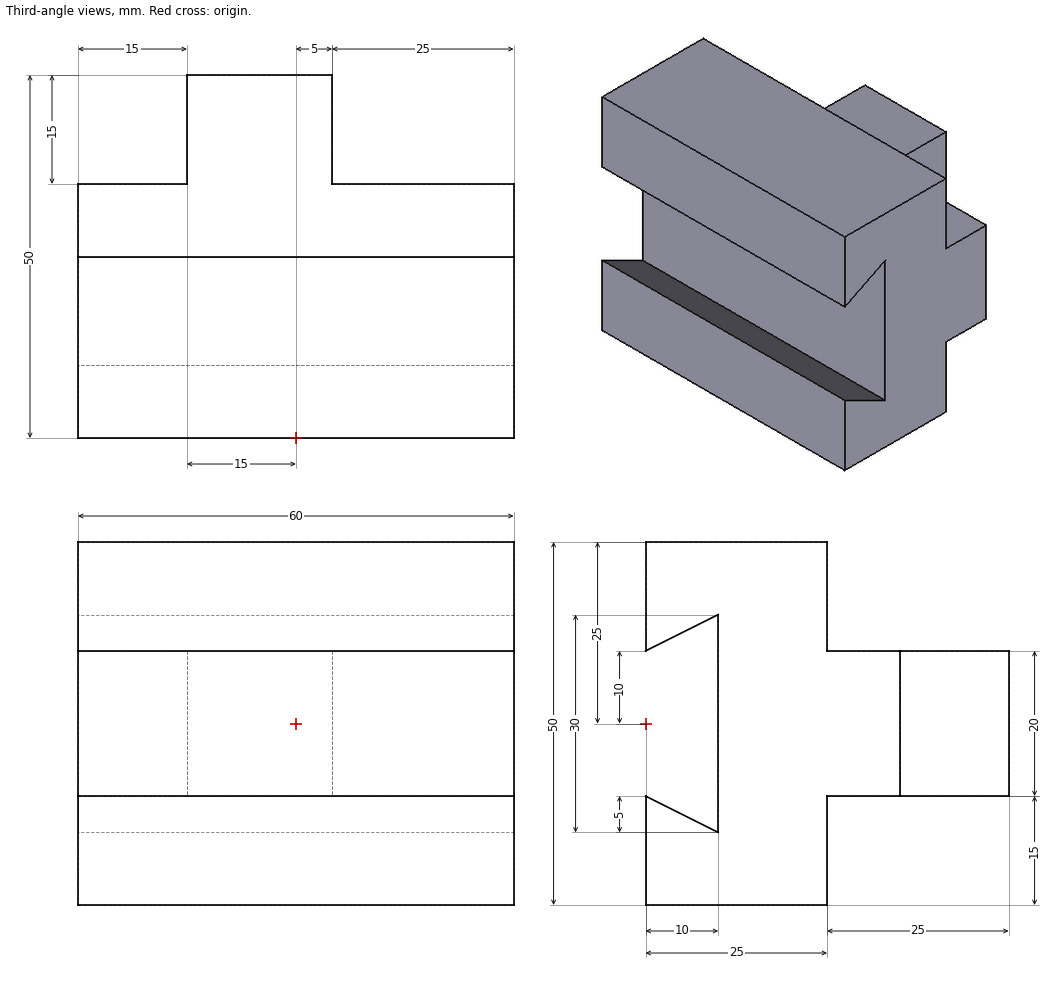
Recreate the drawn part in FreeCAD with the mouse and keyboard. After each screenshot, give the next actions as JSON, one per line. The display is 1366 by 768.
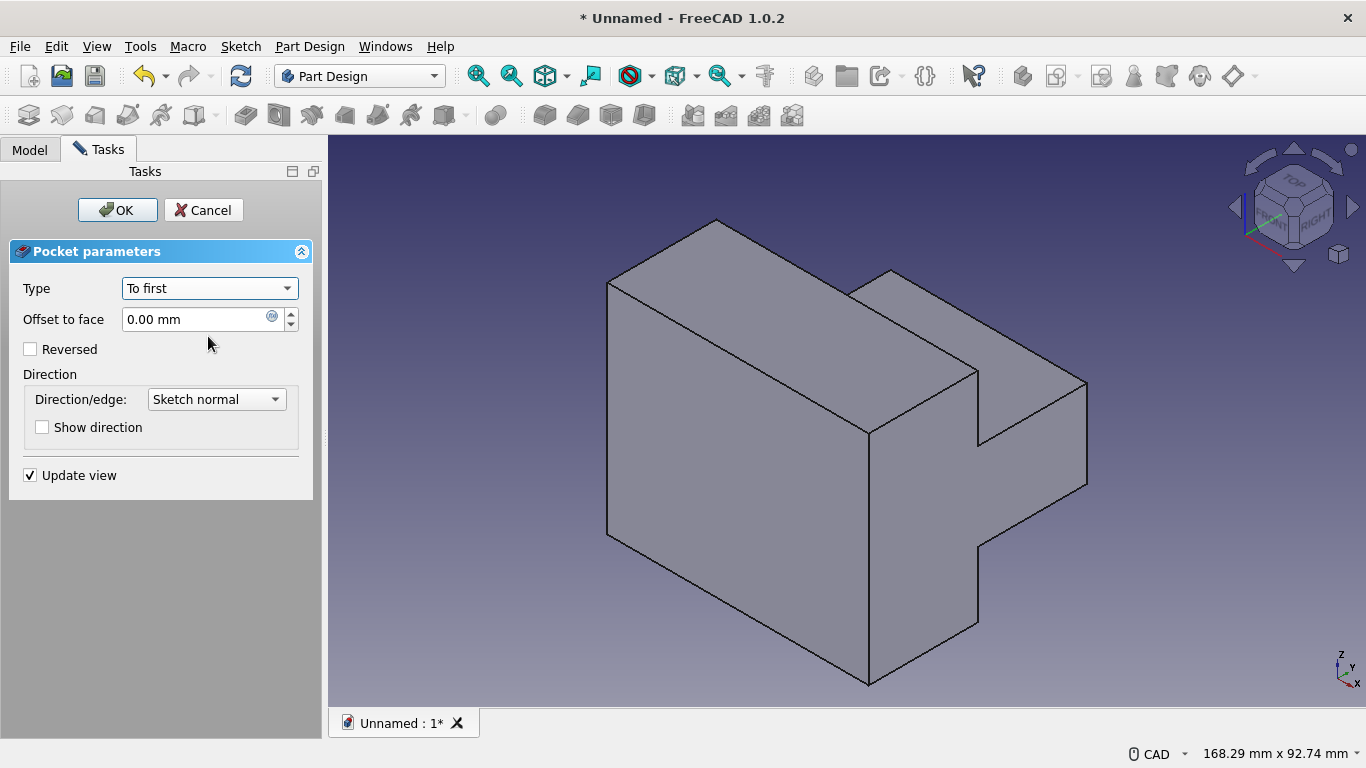
{"action": "left_click", "coordinate": [118, 210]}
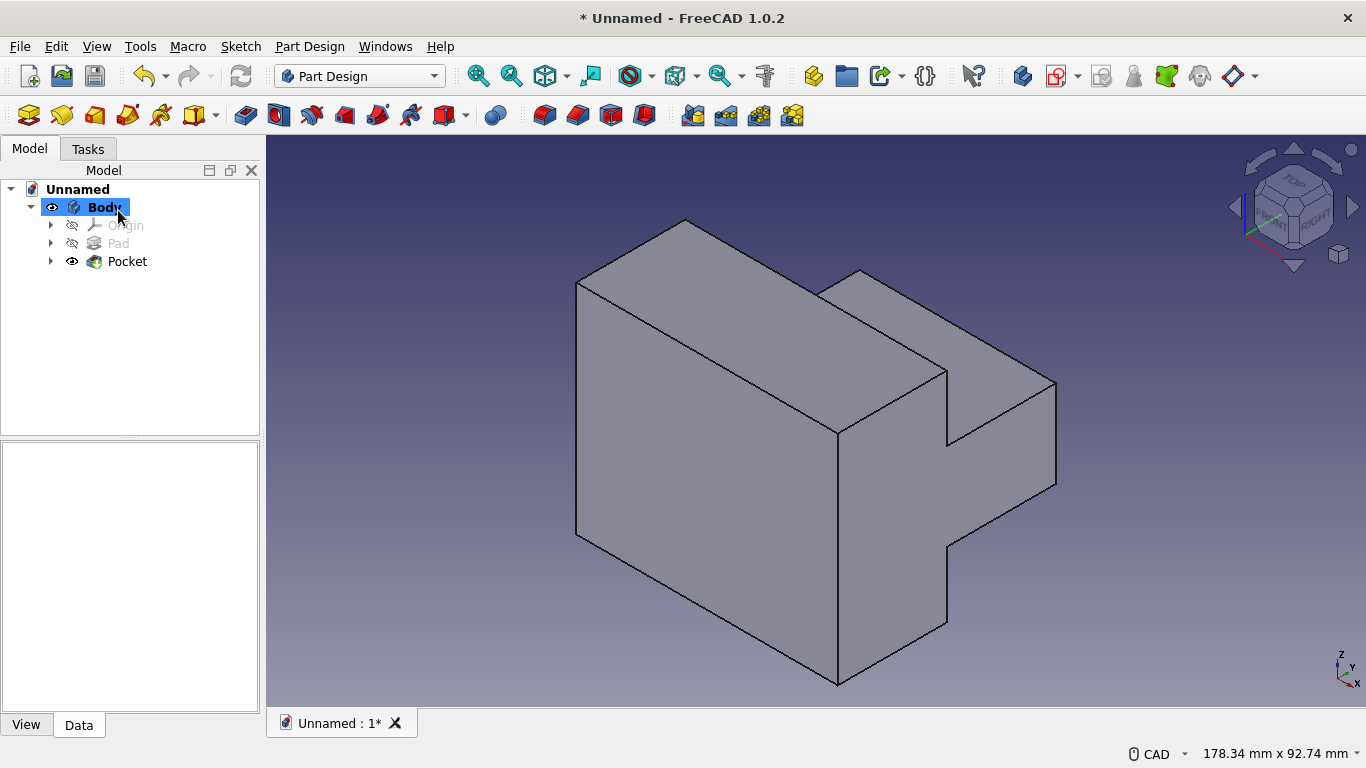
{"action": "left_click", "coordinate": [961, 372]}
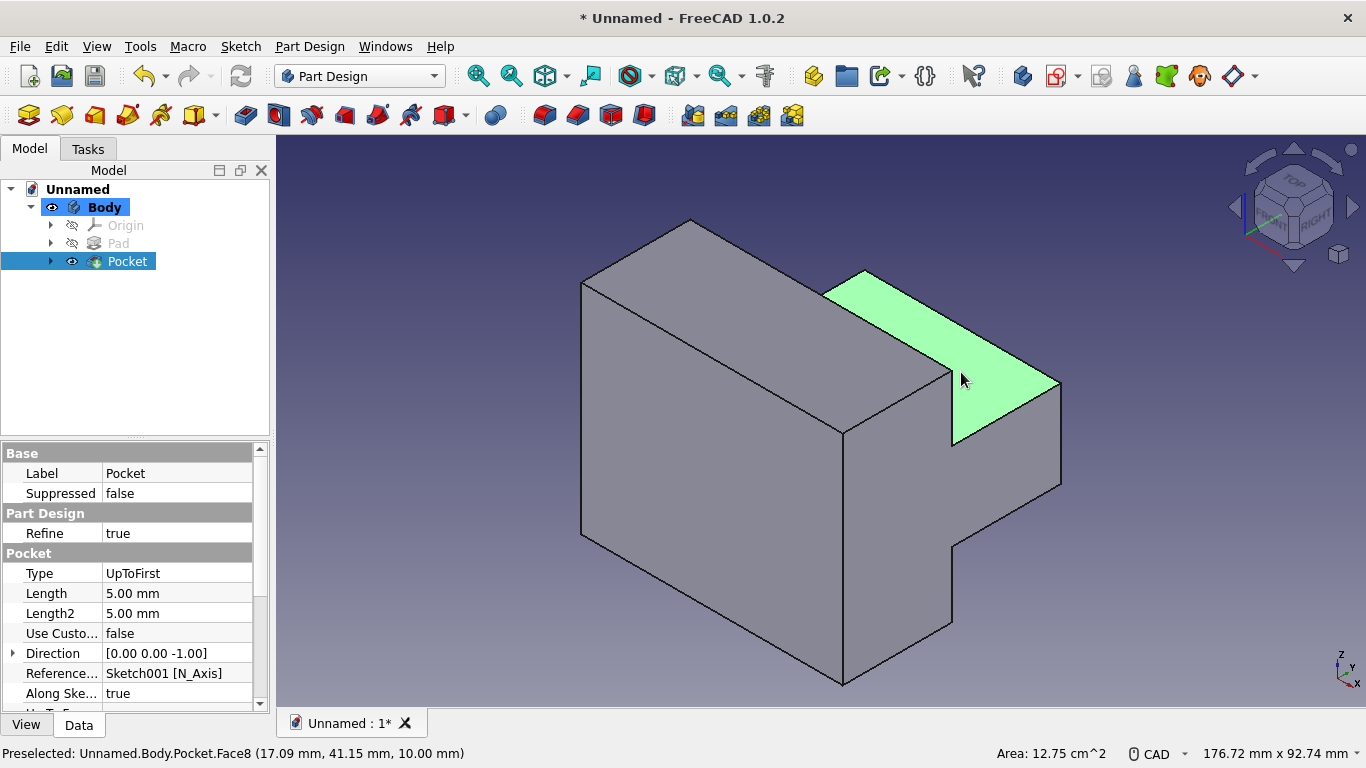
{"action": "left_click", "coordinate": [1056, 76]}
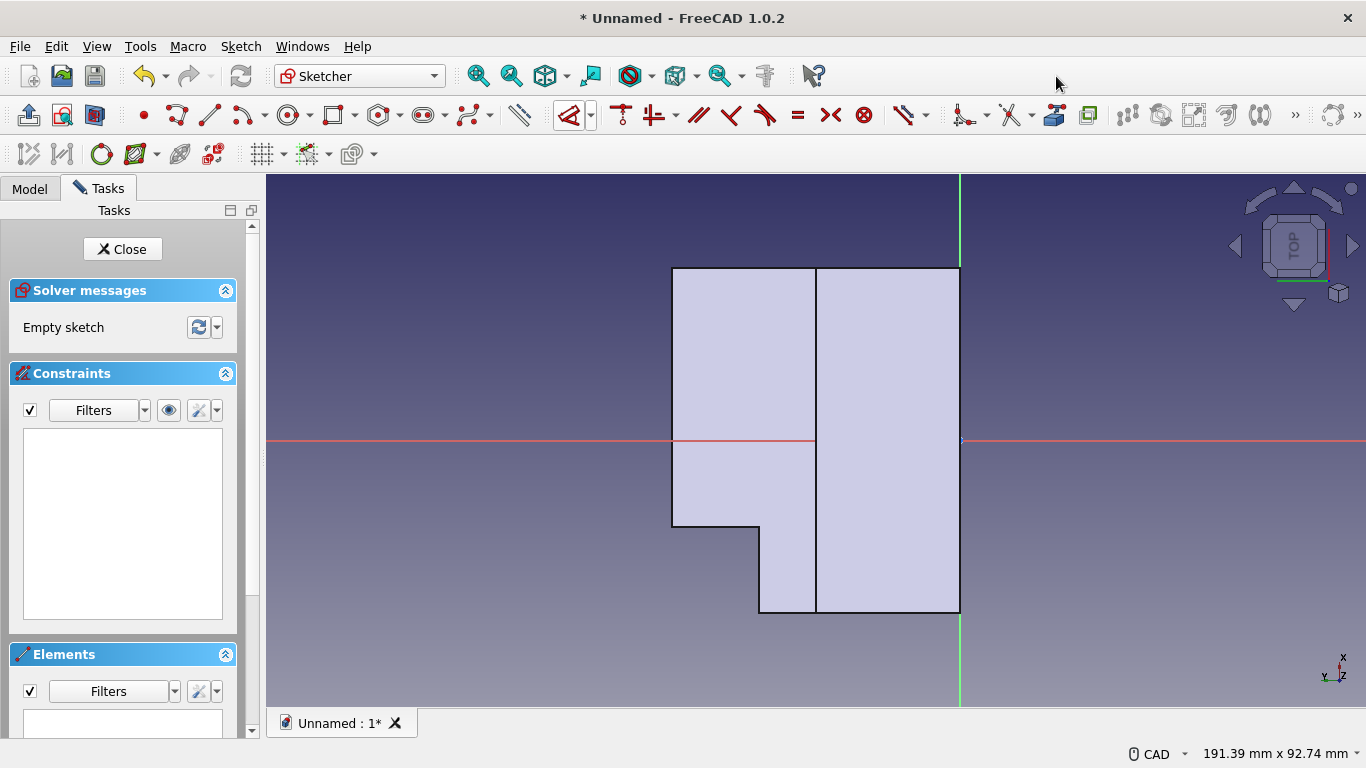
{"action": "key", "text": "q s"}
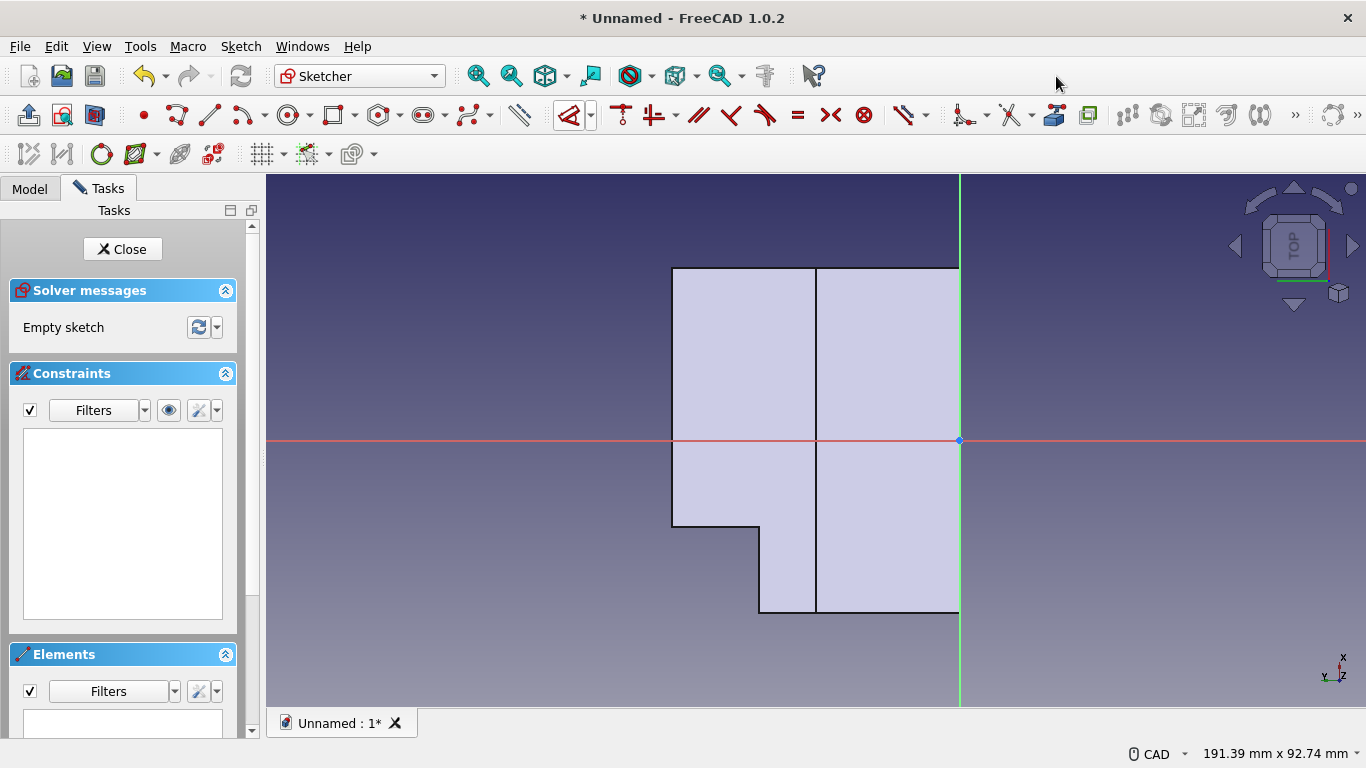
{"action": "scroll", "coordinate": [899, 249], "scroll_direction": "up", "scroll_amount": 3}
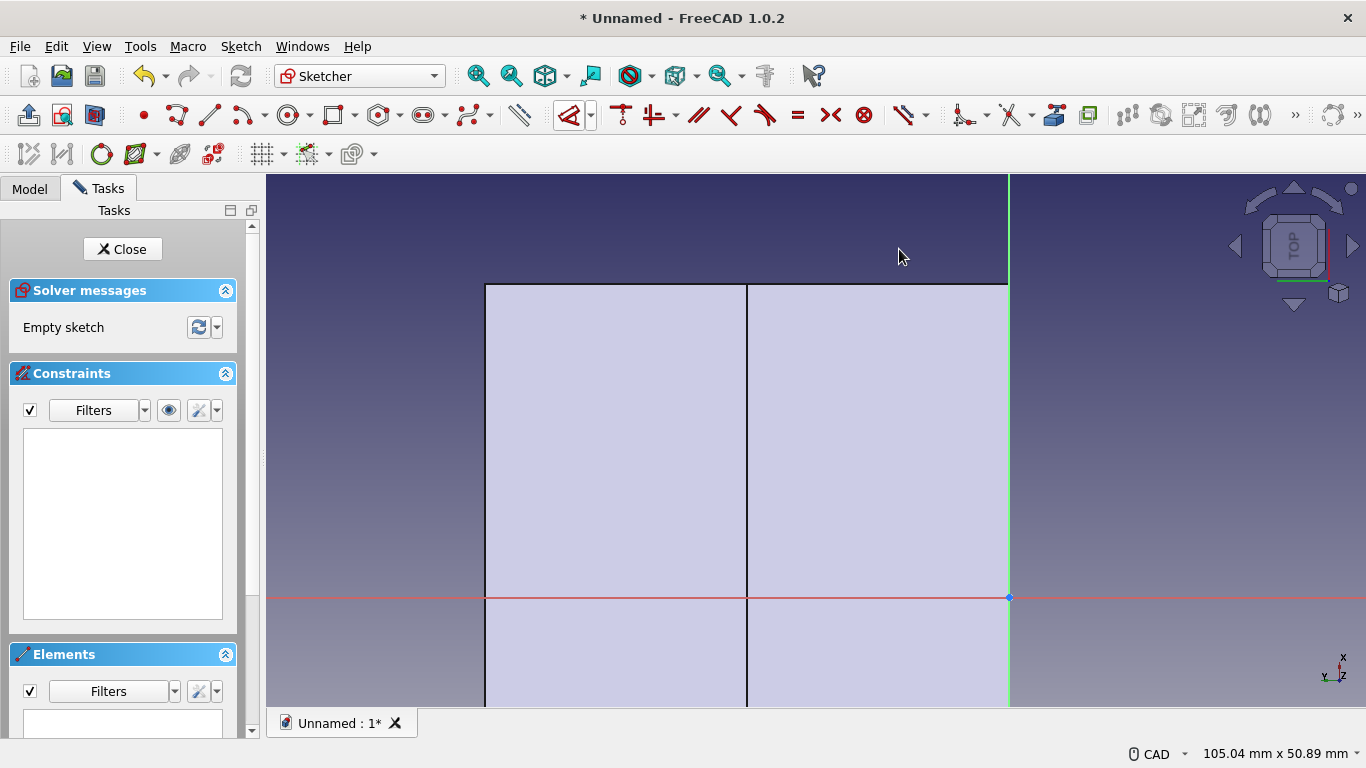
{"action": "key", "text": "g r"}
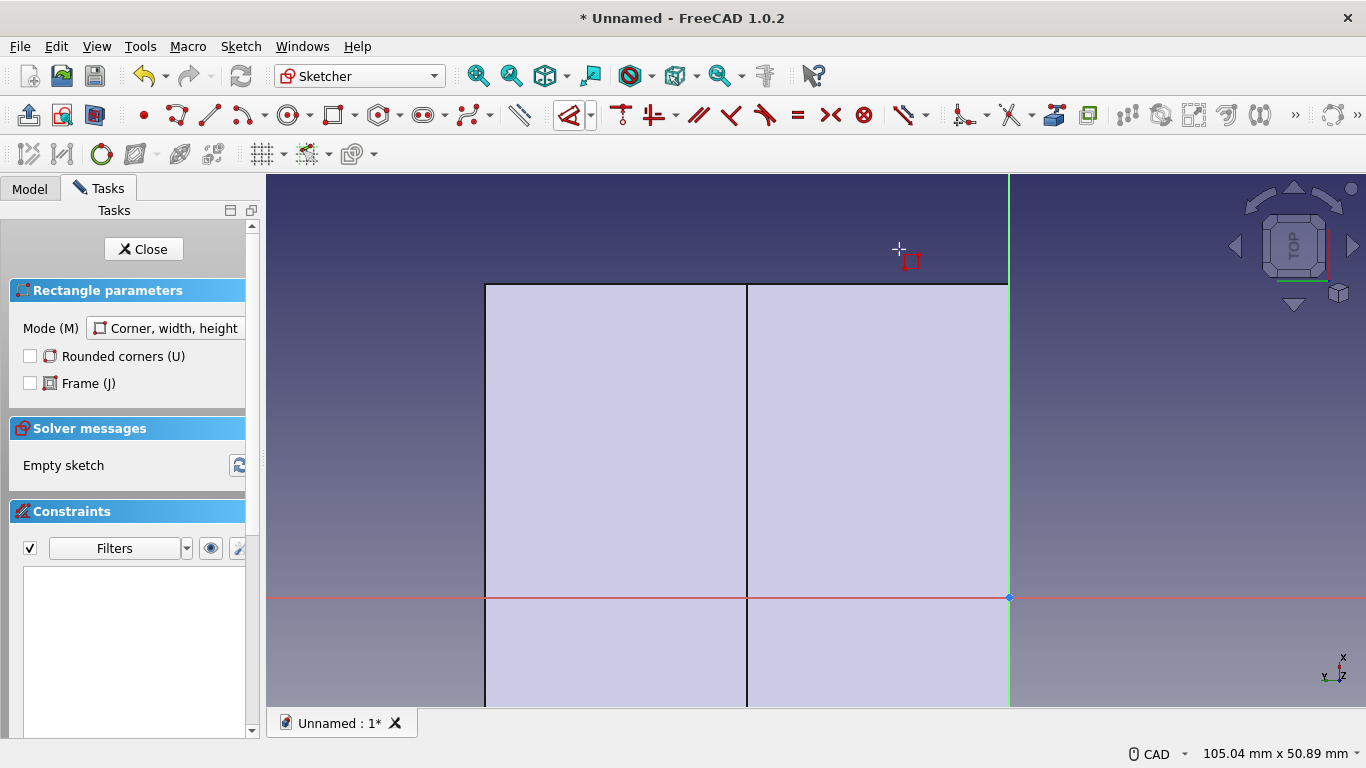
{"action": "left_click", "coordinate": [485, 284]}
{"action": "mouse_move", "coordinate": [643, 545]}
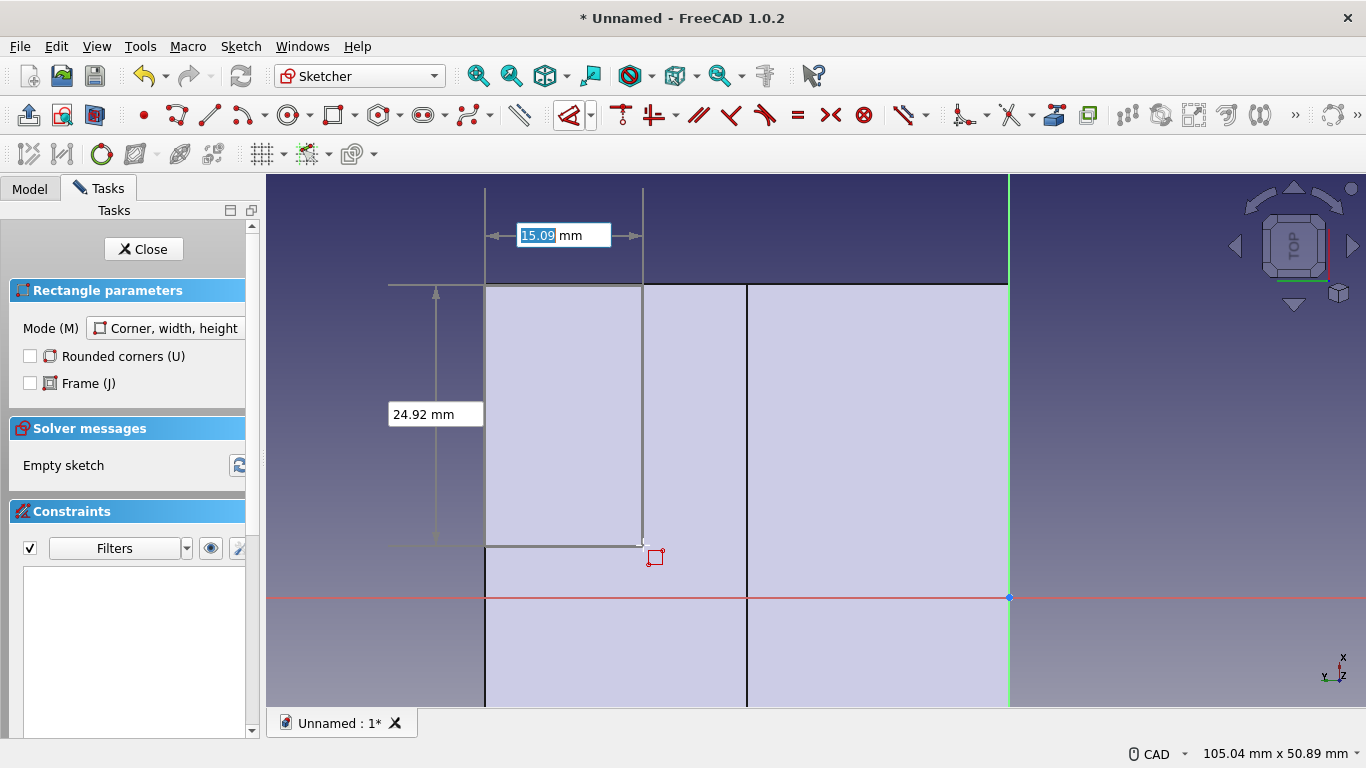
{"action": "type", "text": "15"}
{"action": "key", "text": "Tab"}
{"action": "type", "text": "25"}
{"action": "key", "text": "Return"}
{"action": "key", "text": "Escape"}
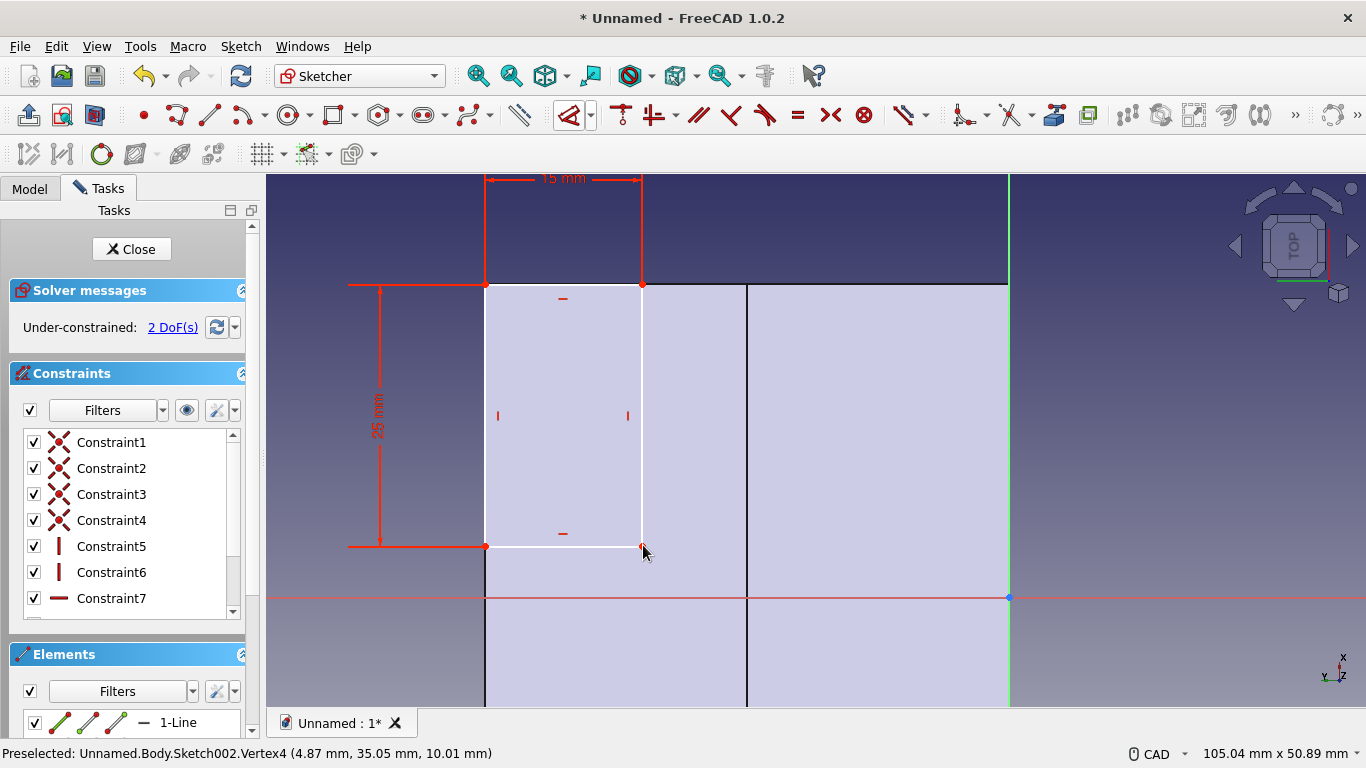
{"action": "left_click", "coordinate": [485, 547]}